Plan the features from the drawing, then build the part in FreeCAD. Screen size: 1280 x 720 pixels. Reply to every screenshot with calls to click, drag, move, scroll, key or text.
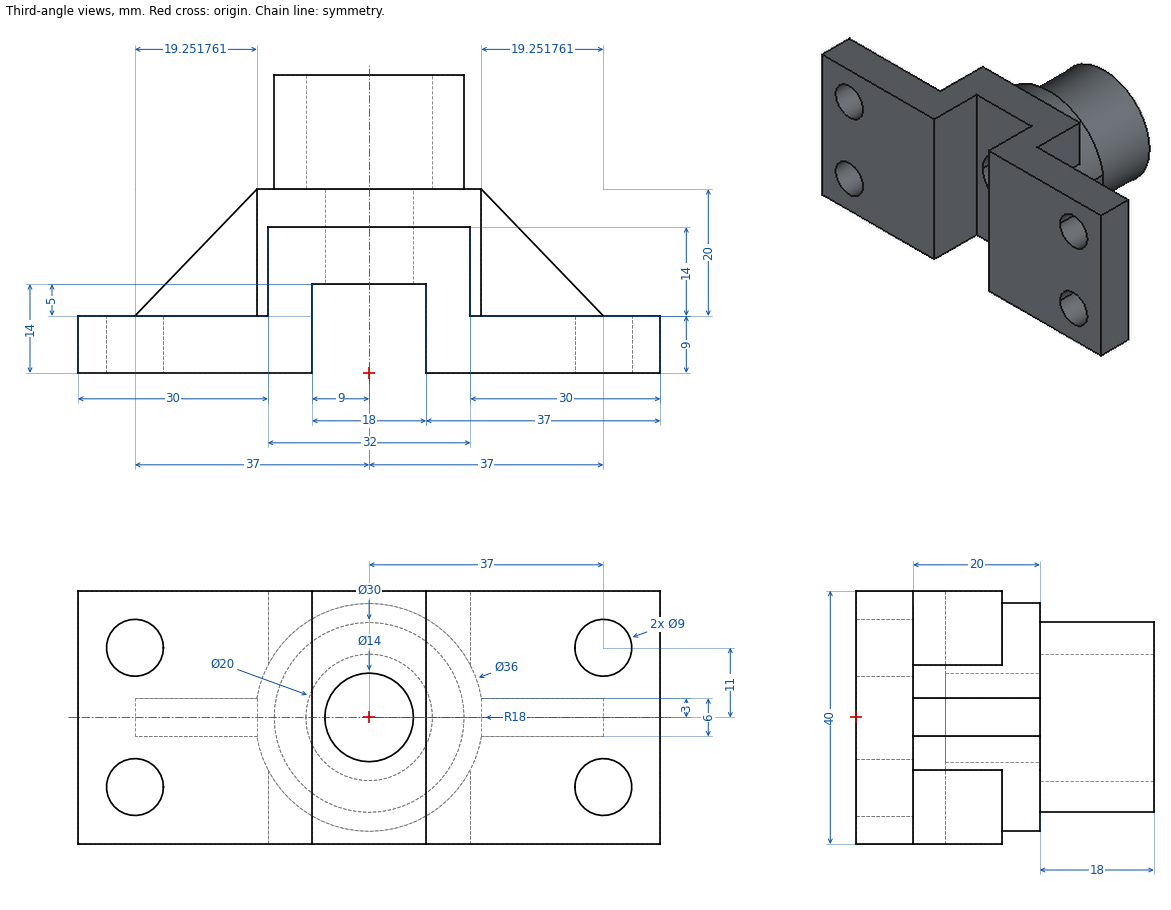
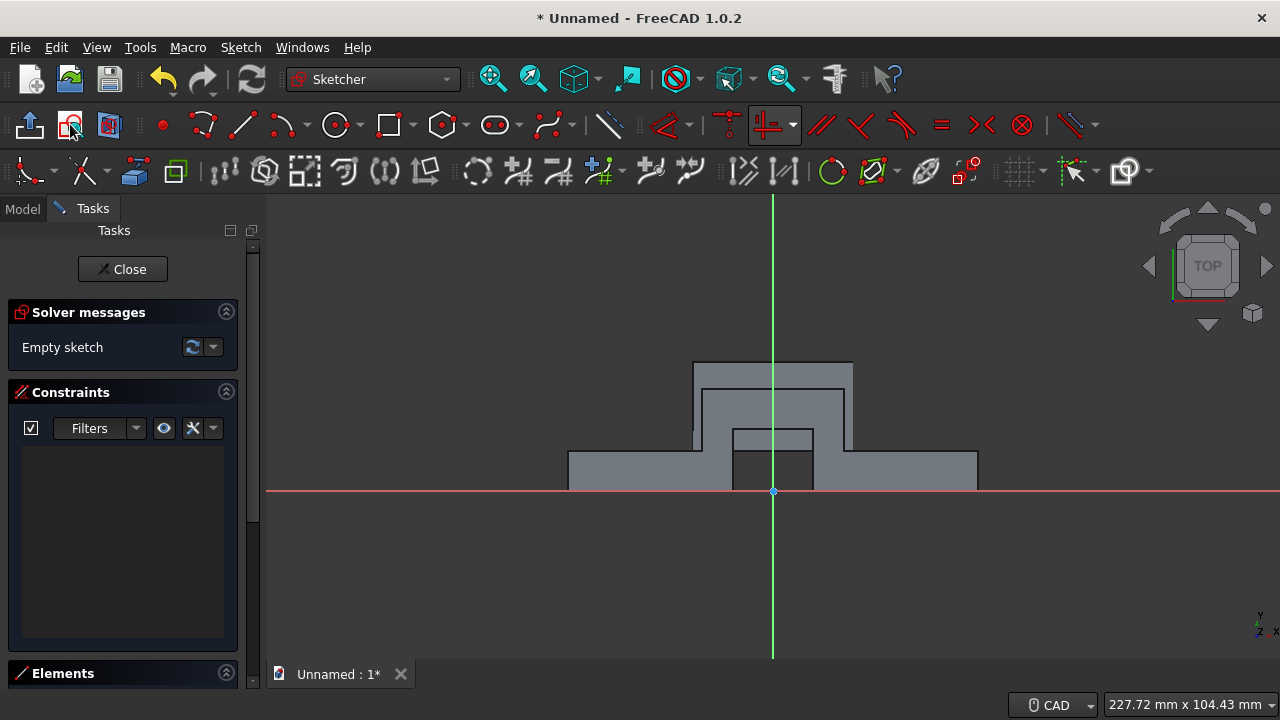
scroll(790, 468, up, 8)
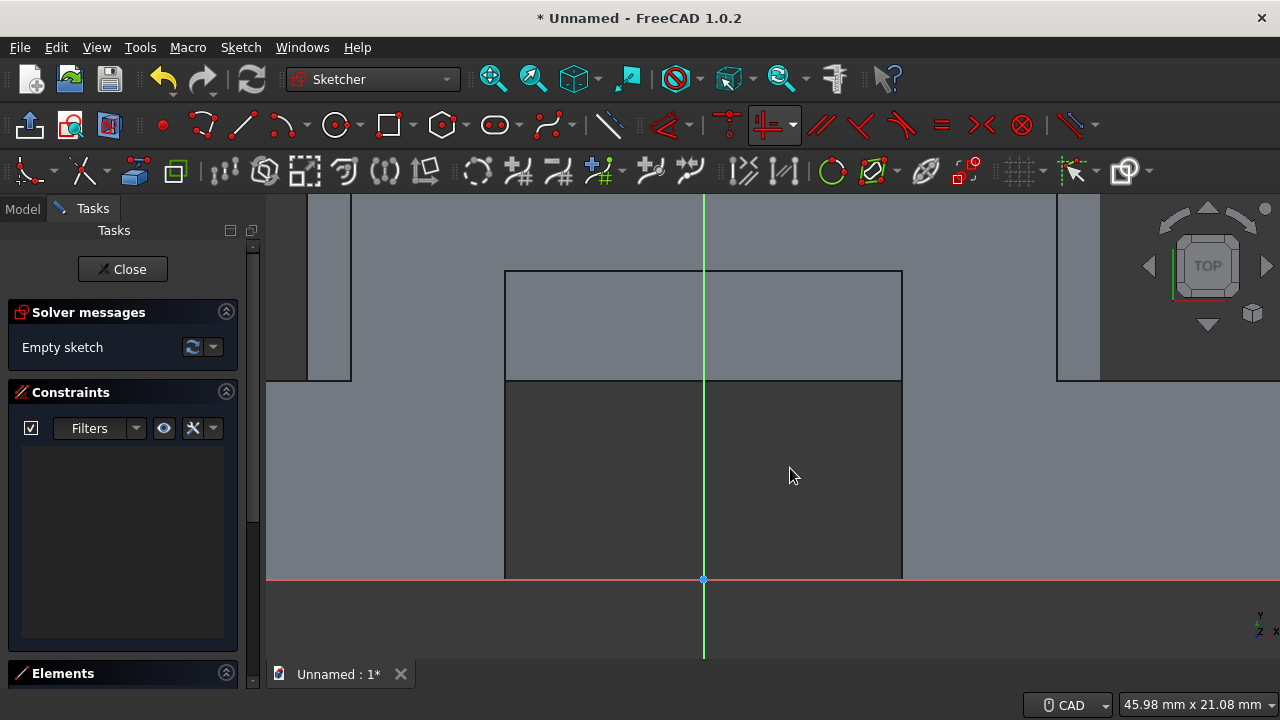
click(390, 126)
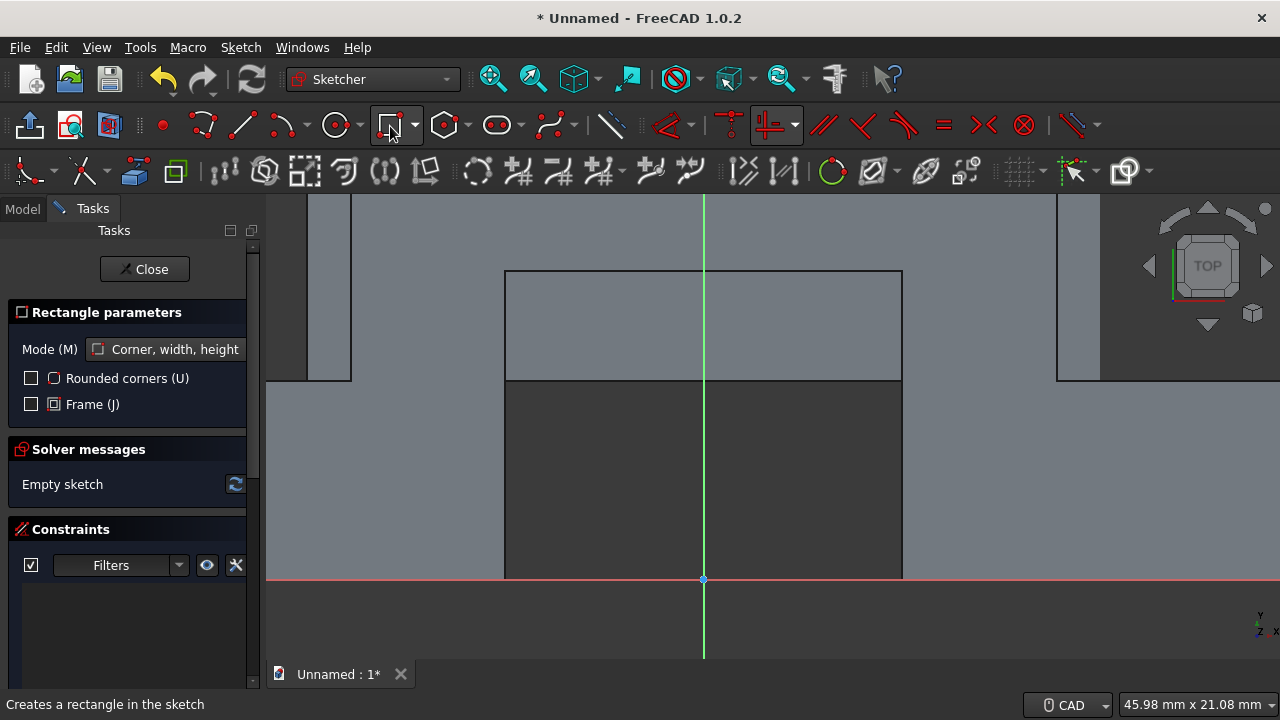
click(505, 271)
click(902, 381)
key(Escape)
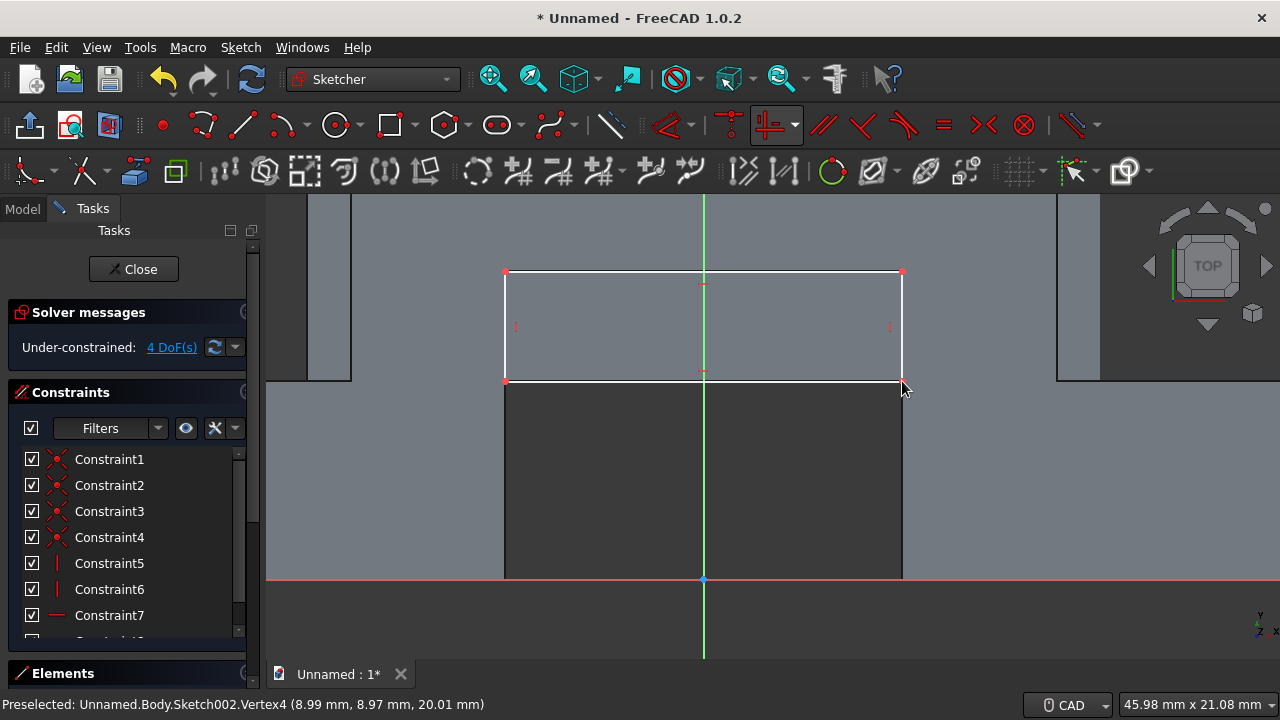
key(d)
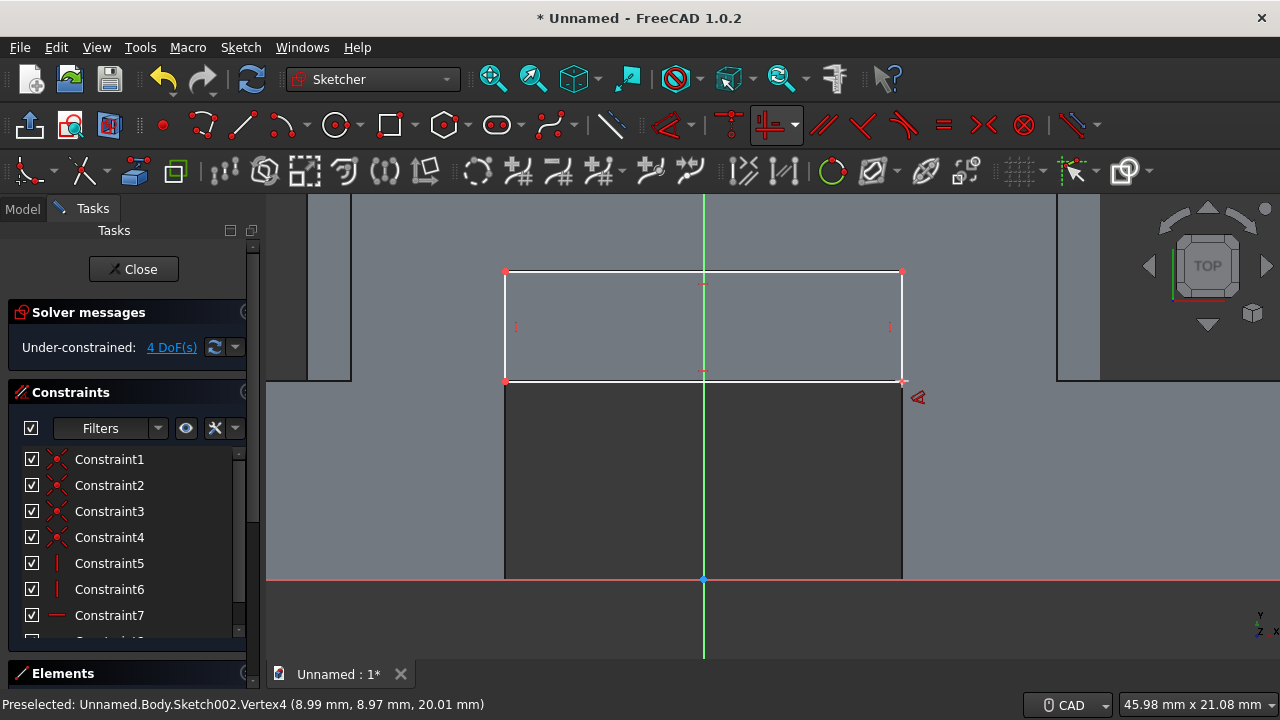
click(505, 305)
click(471, 327)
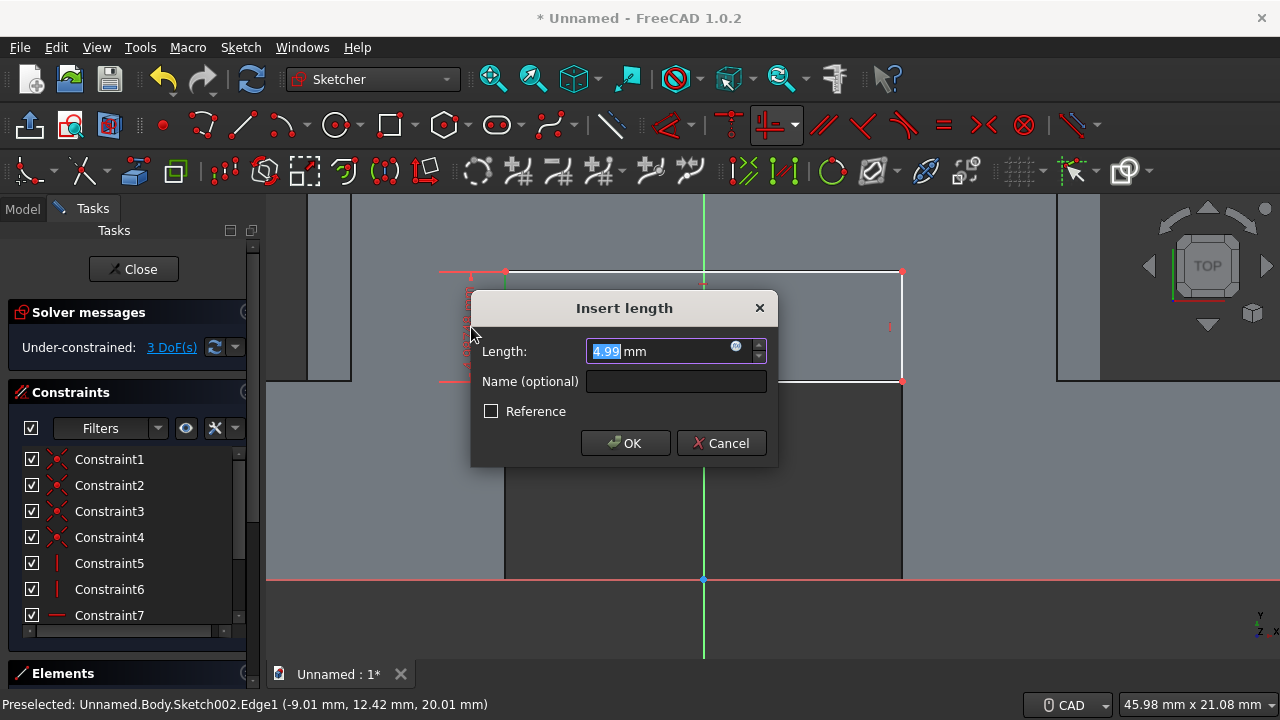
text(5)
key(Return)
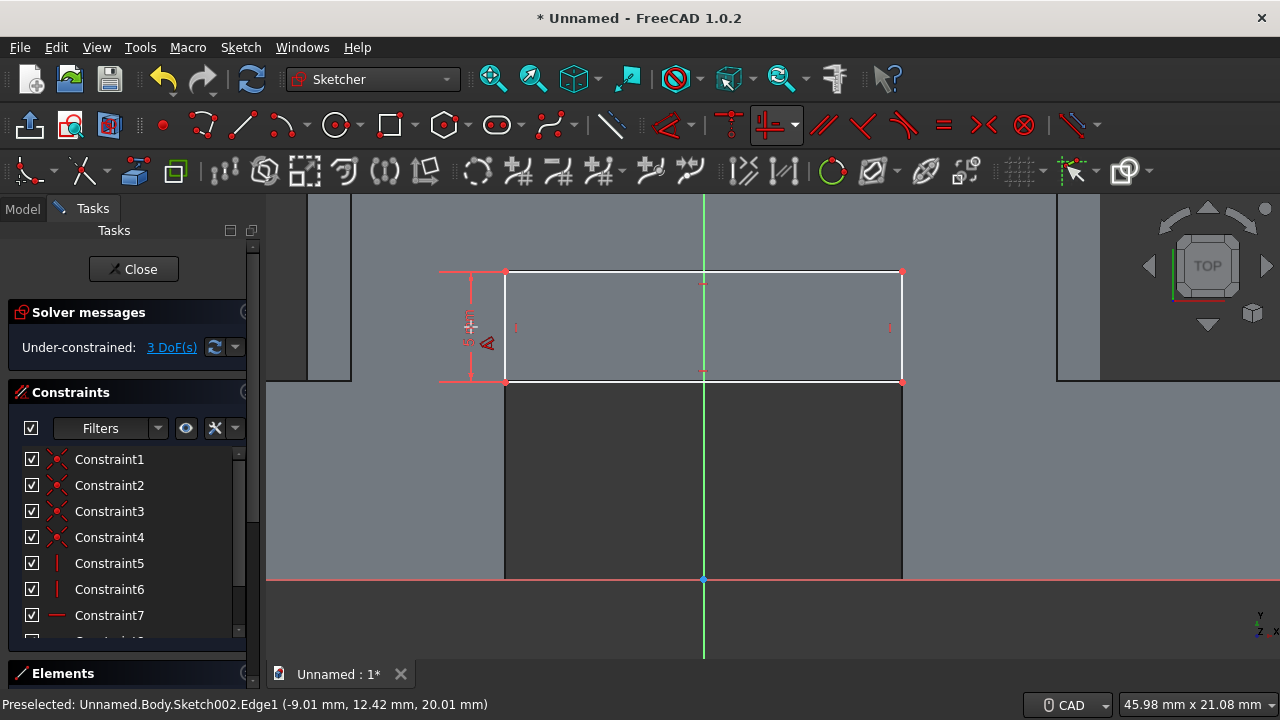
click(624, 382)
click(612, 348)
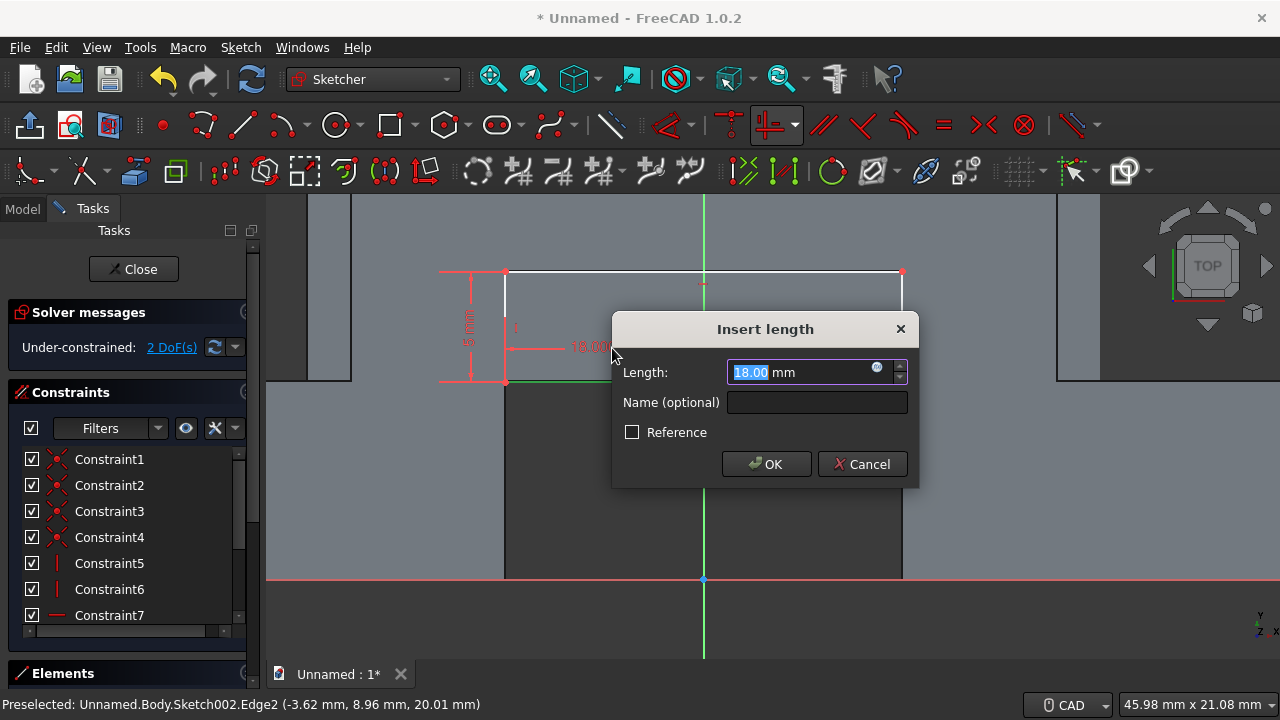
text(18)
key(Return)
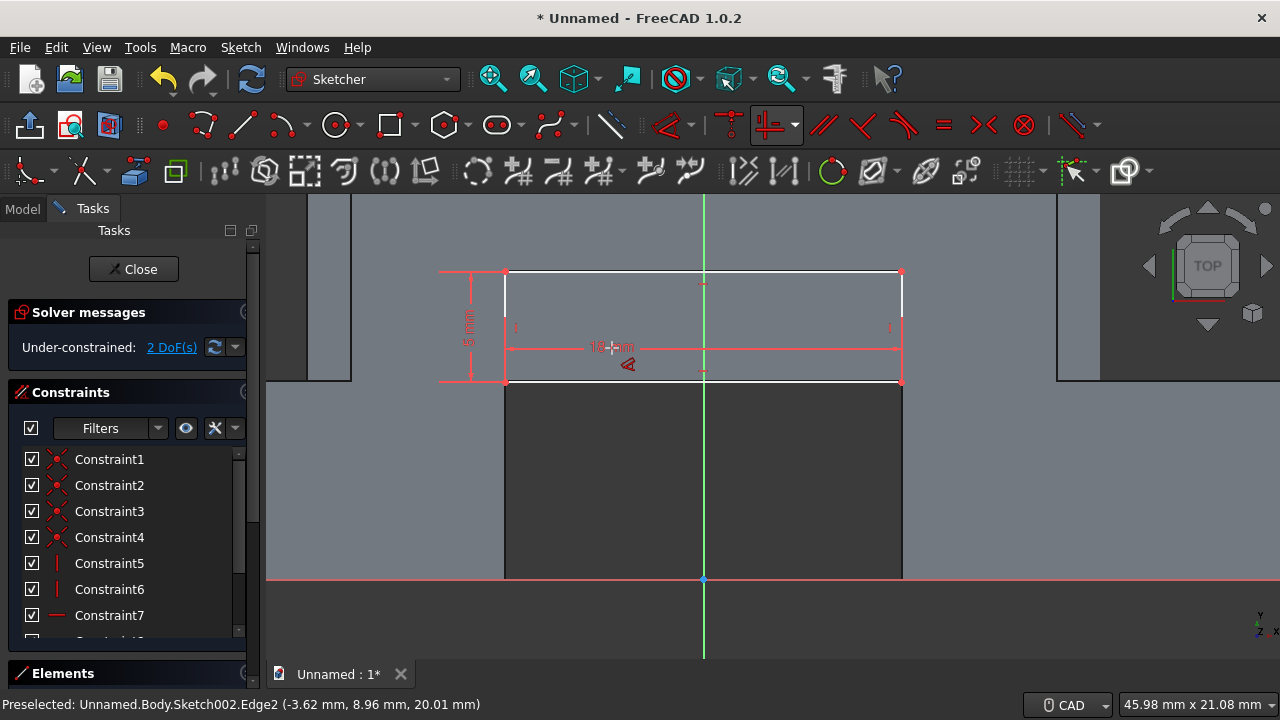
click(505, 272)
click(604, 614)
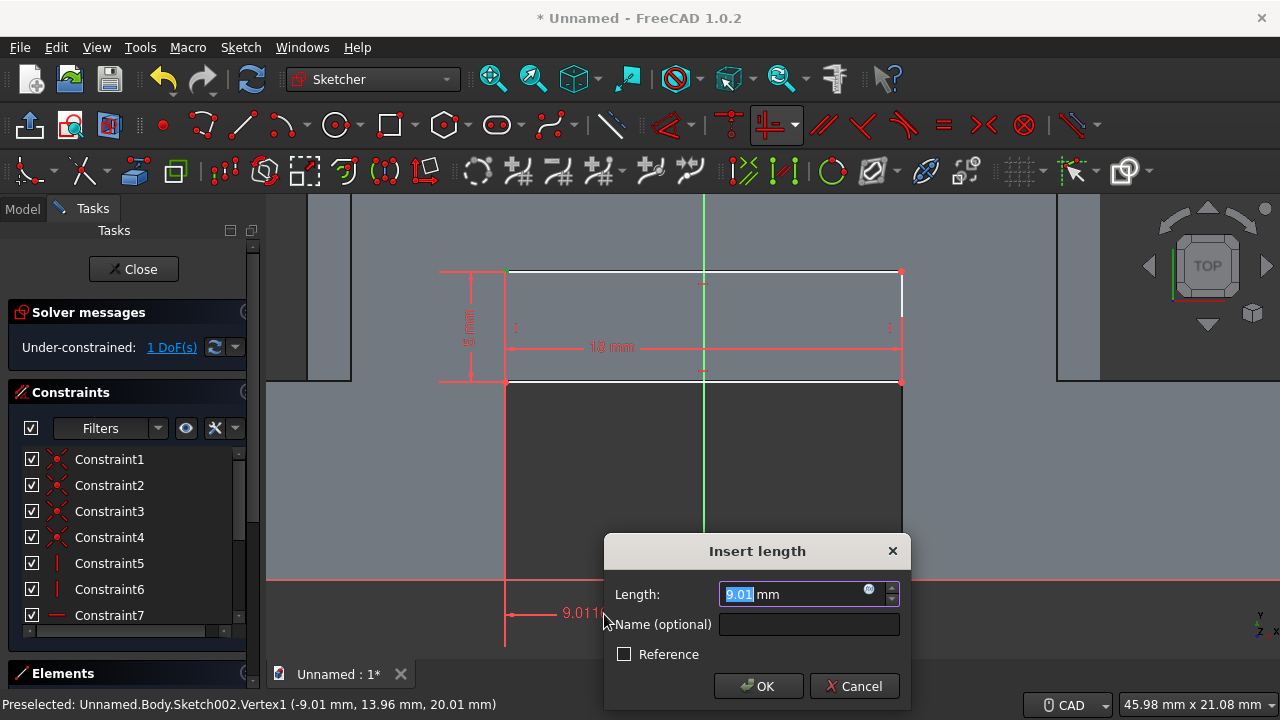
text(9)
key(Return)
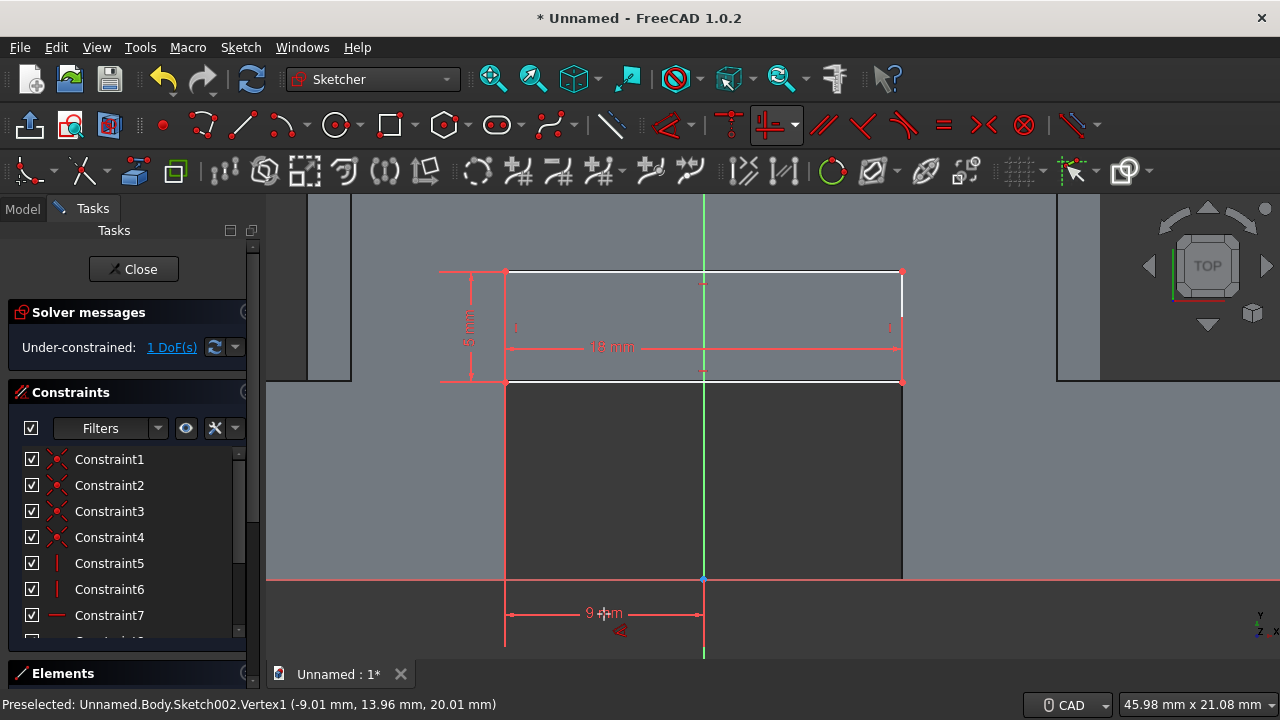
click(505, 382)
click(471, 481)